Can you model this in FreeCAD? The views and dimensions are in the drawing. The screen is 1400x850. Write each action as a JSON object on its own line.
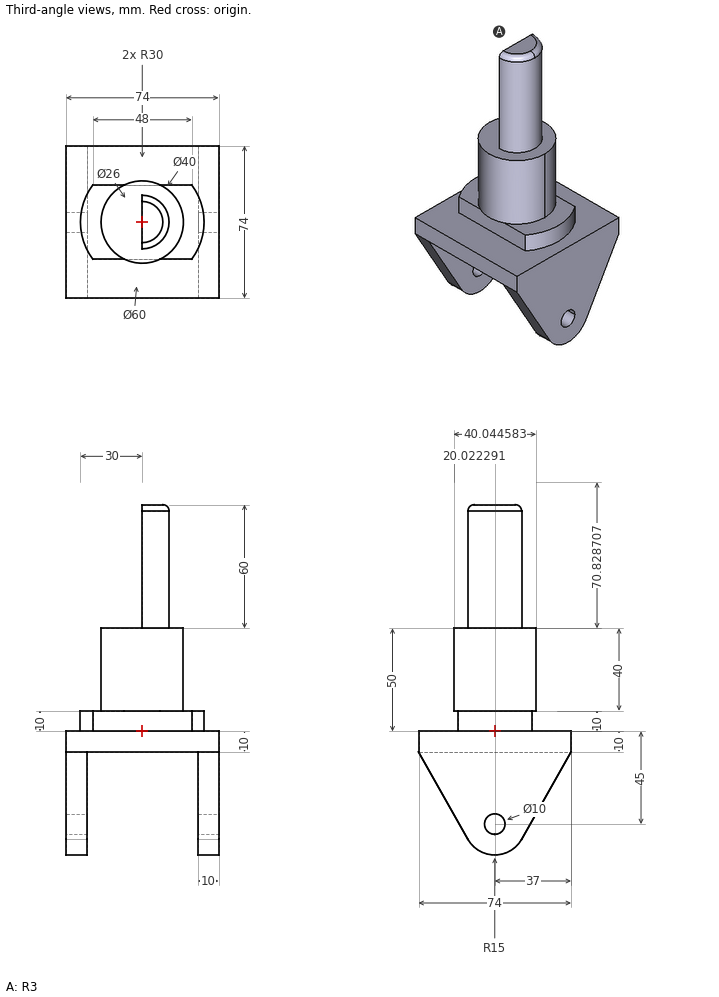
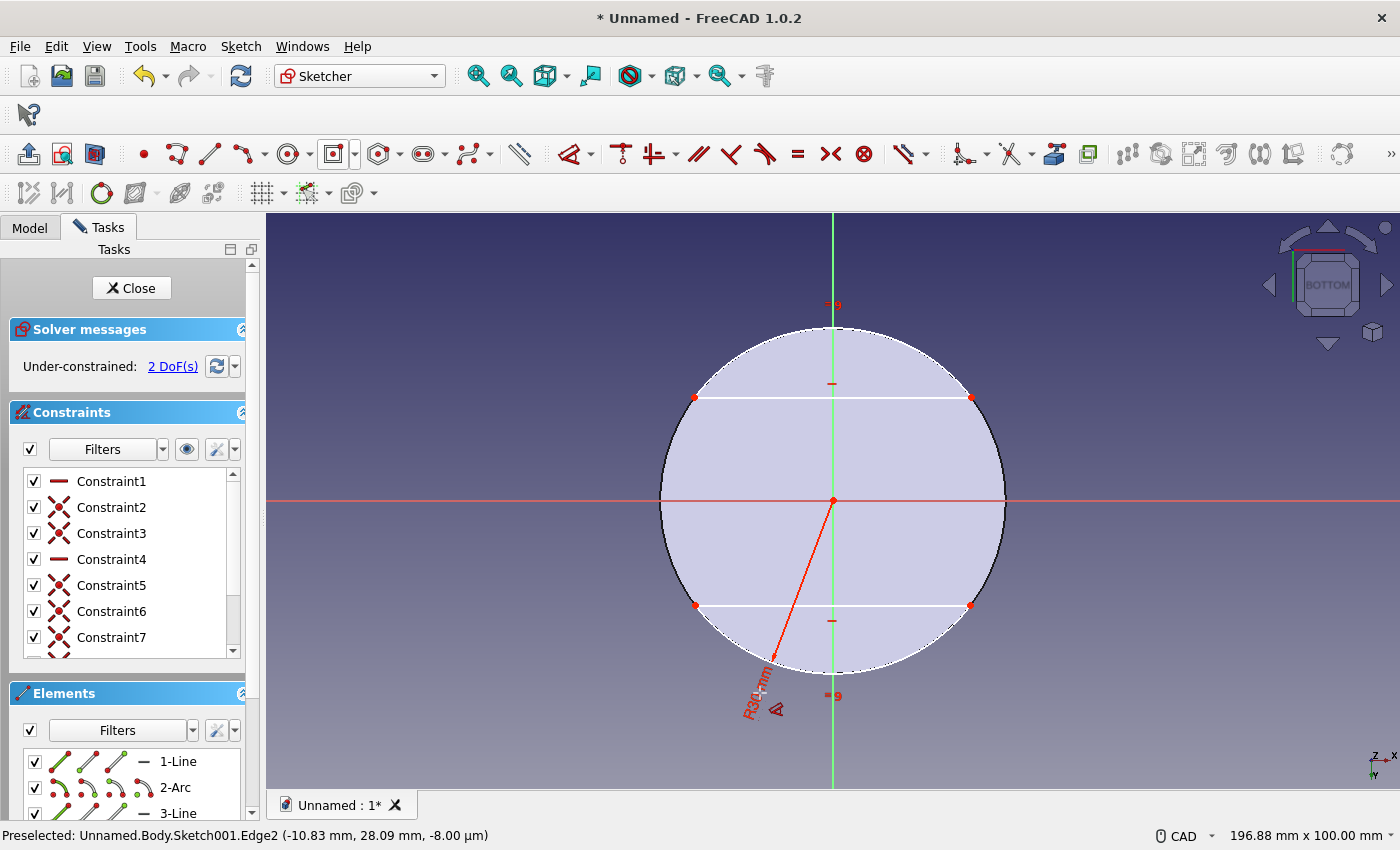
{"action": "left_click", "coordinate": [888, 606]}
{"action": "left_click", "coordinate": [770, 640]}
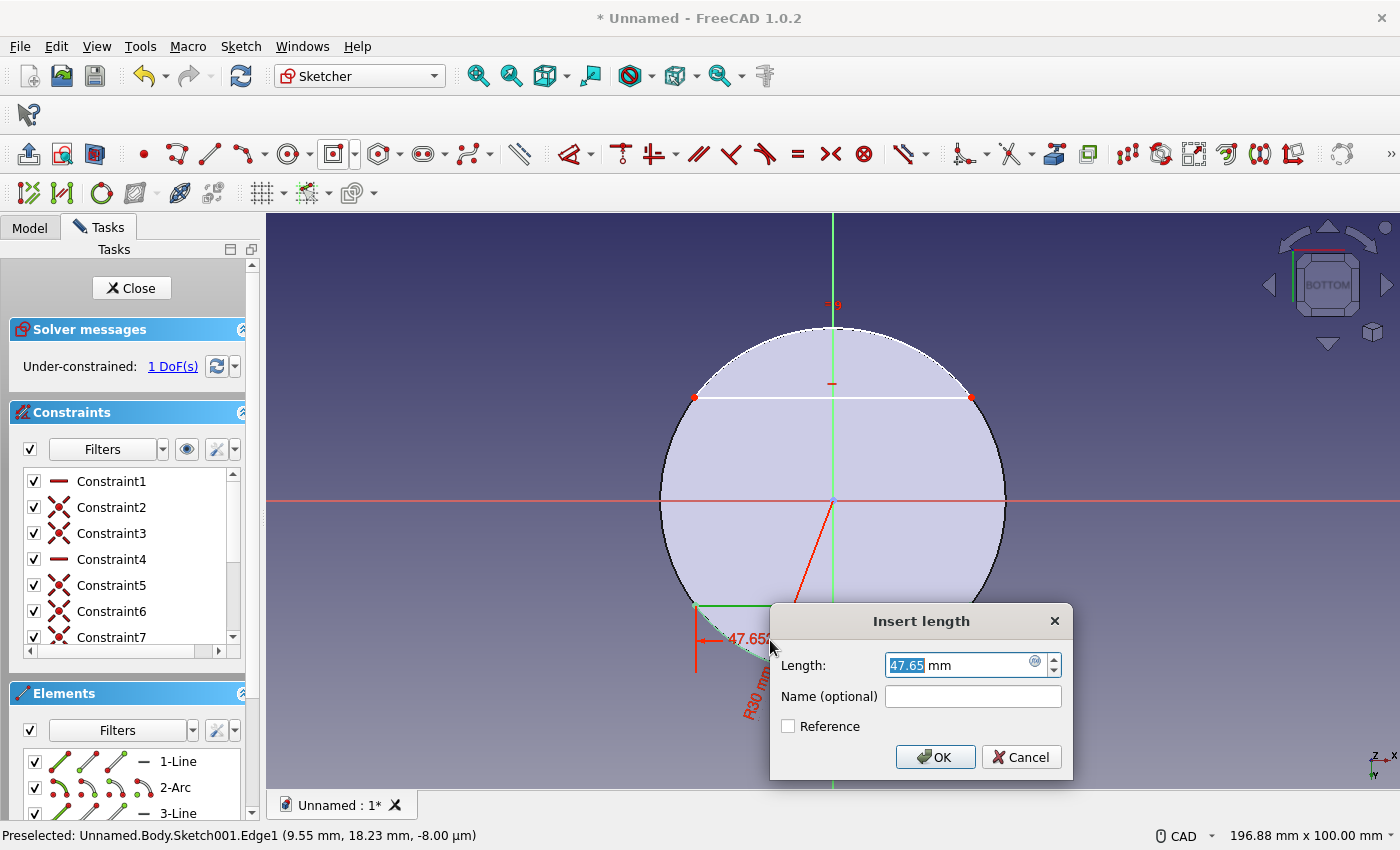
{"action": "type", "text": "48"}
{"action": "key", "text": "Return"}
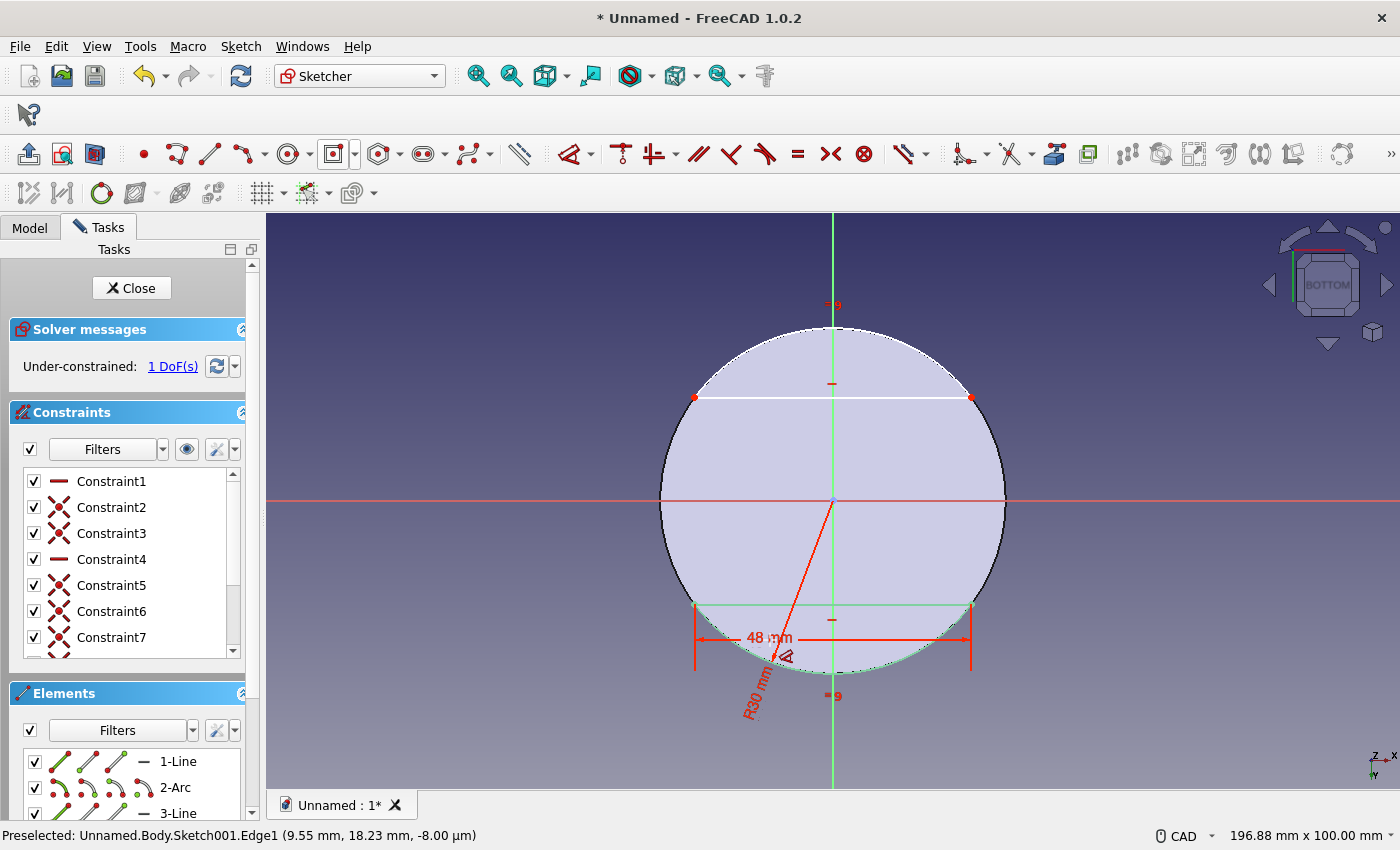
{"action": "left_click", "coordinate": [778, 398]}
{"action": "left_click", "coordinate": [769, 364]}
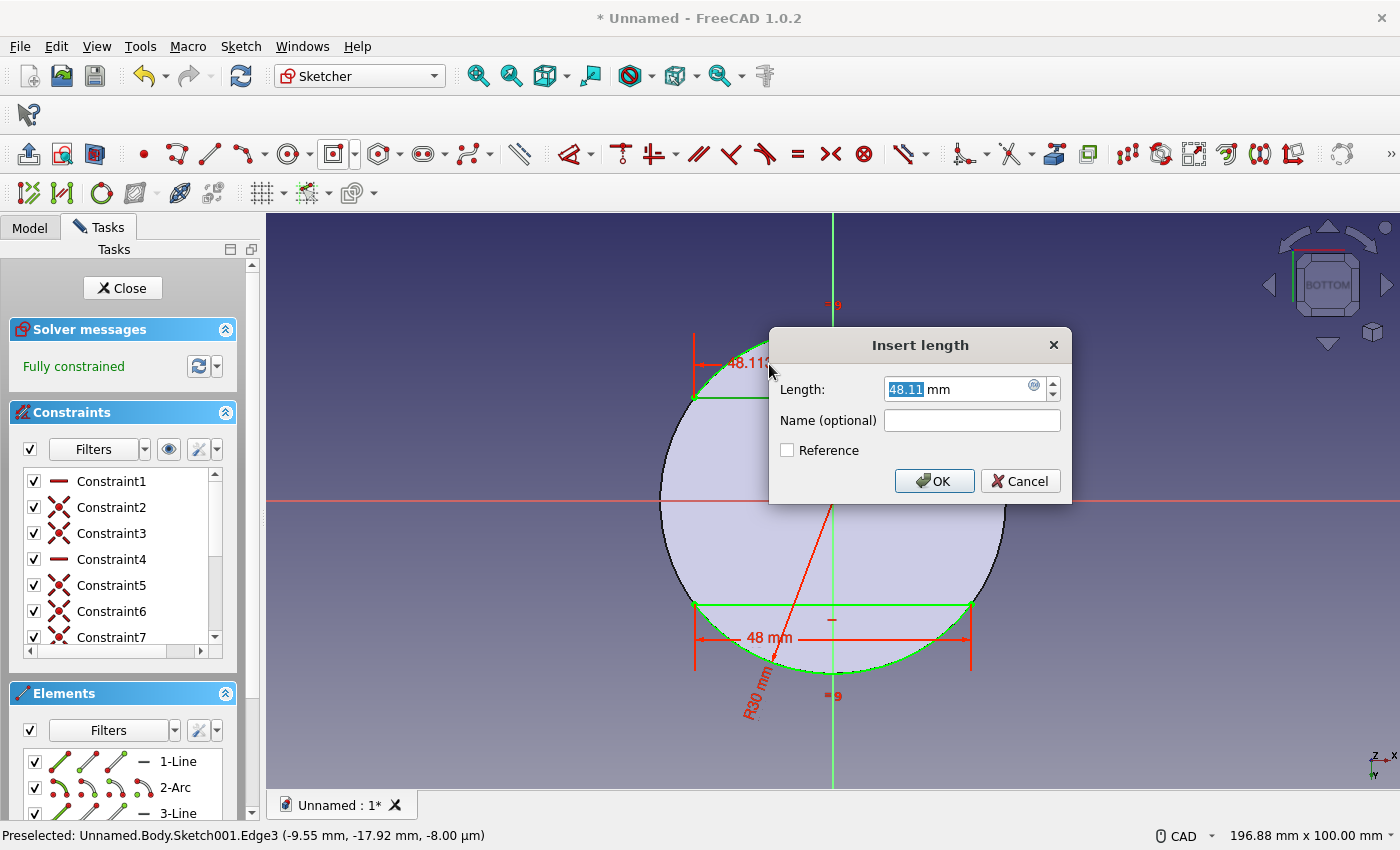
{"action": "type", "text": "48"}
{"action": "key", "text": "Return"}
{"action": "key", "text": "Escape"}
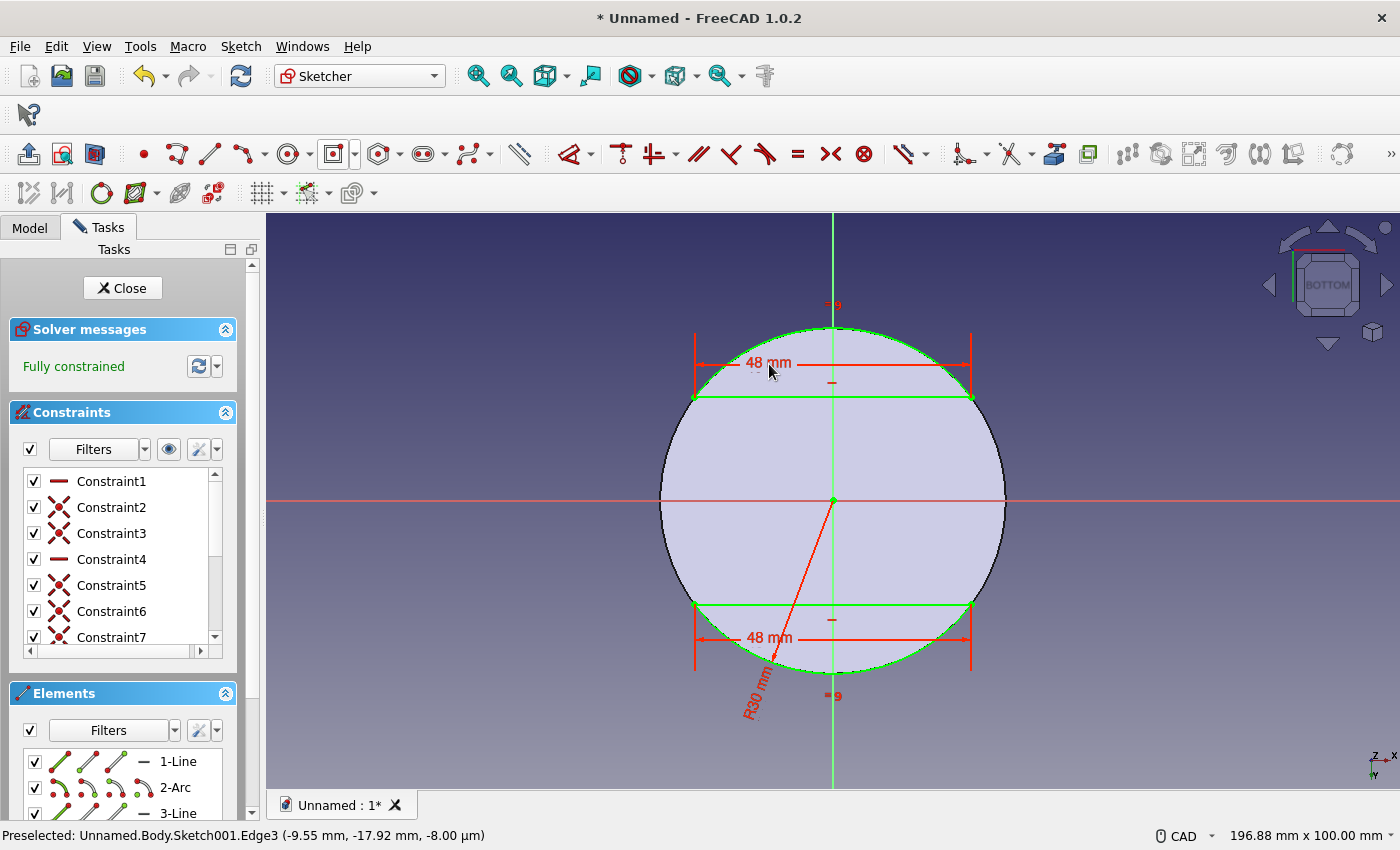
{"action": "left_click", "coordinate": [123, 288]}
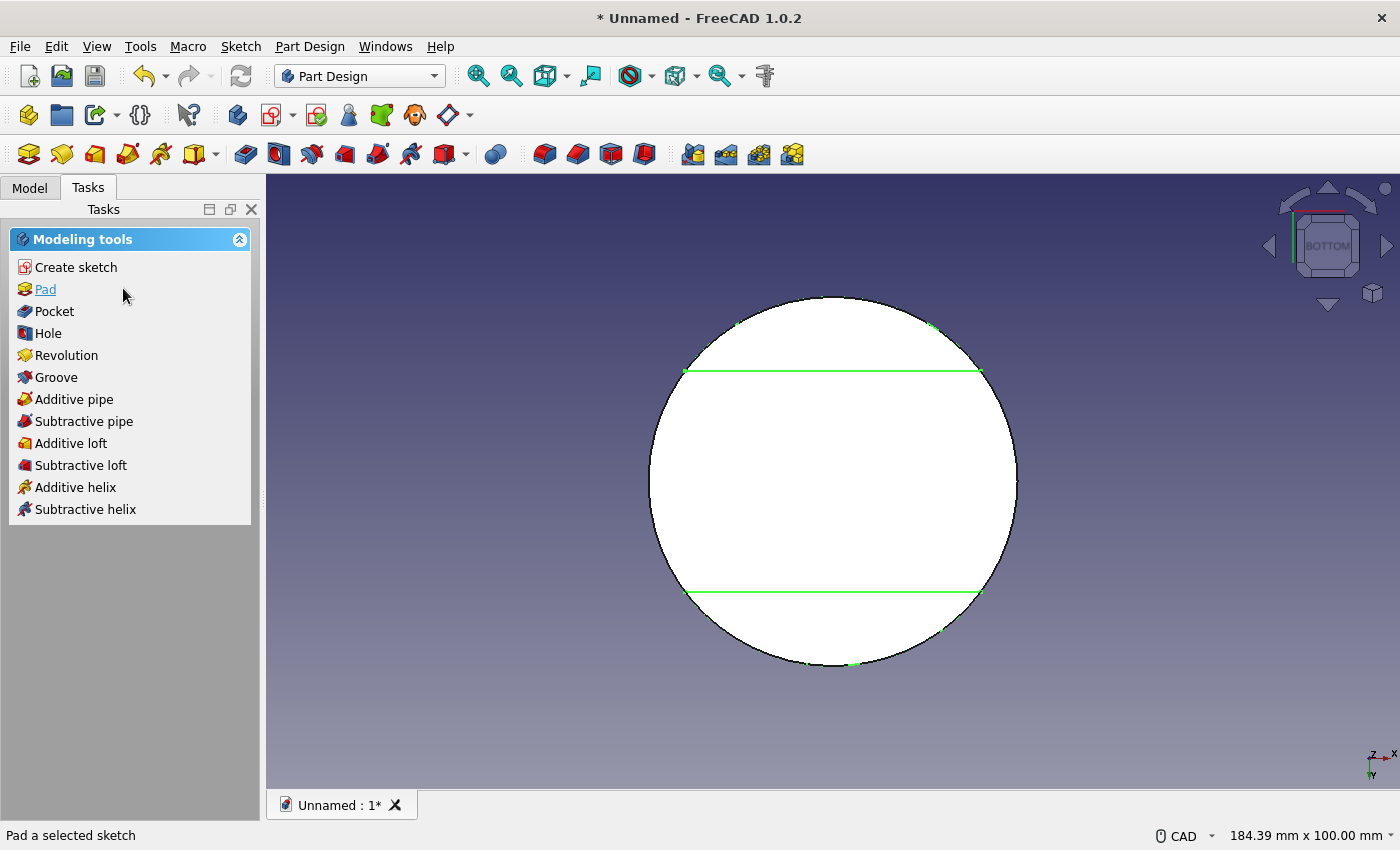
{"action": "left_click", "coordinate": [246, 154]}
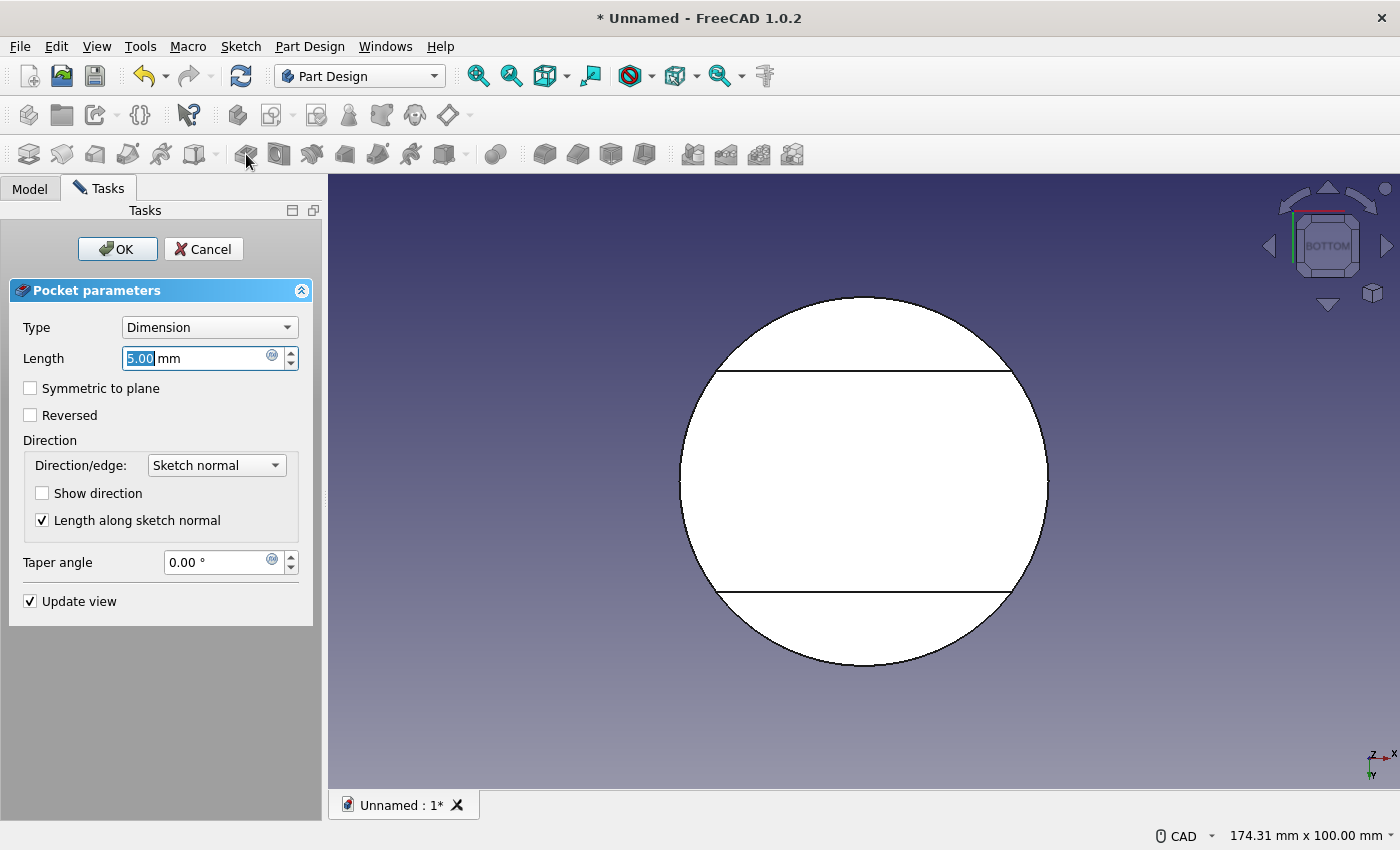
{"action": "type", "text": "10"}
{"action": "key", "text": "Tab"}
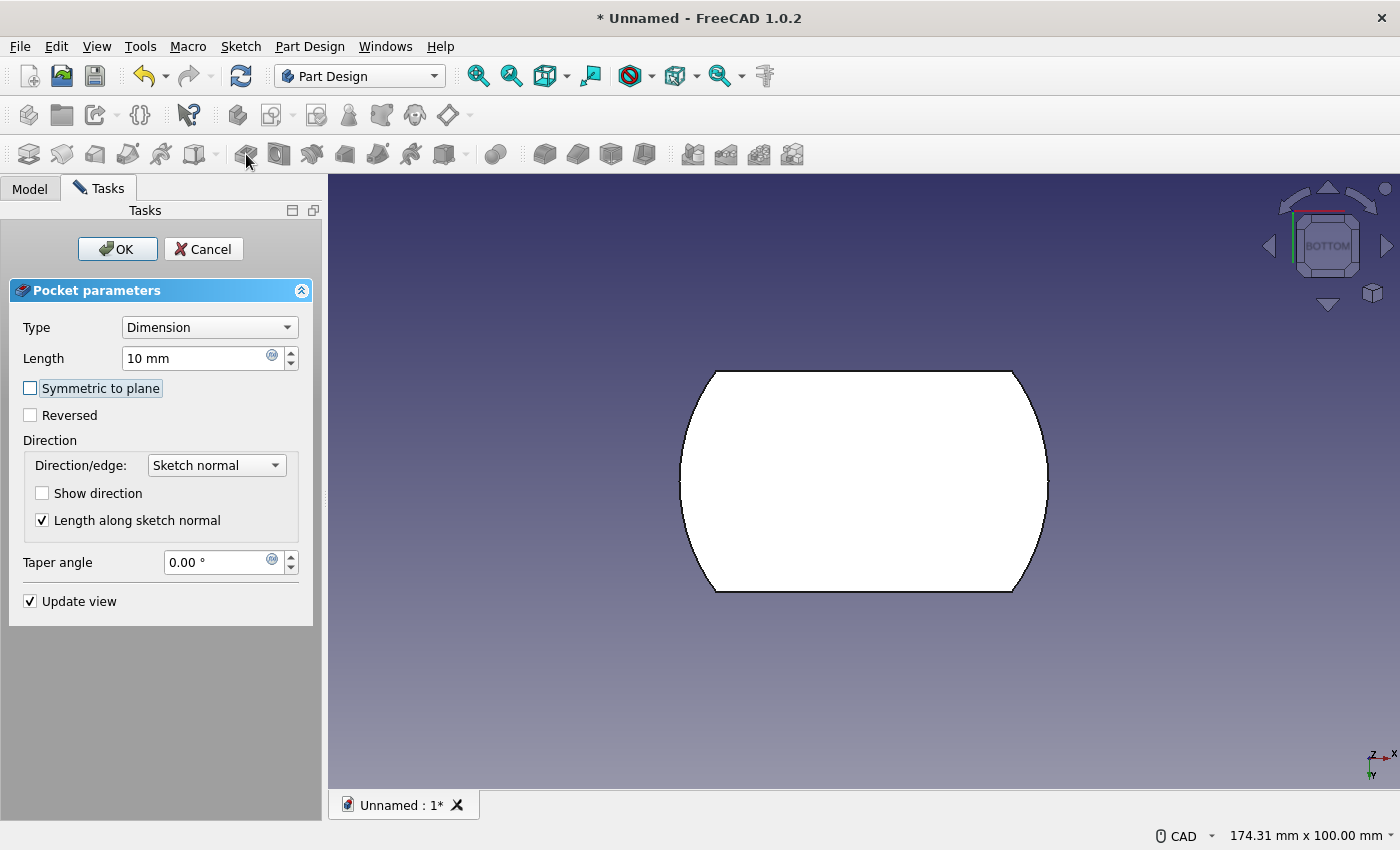
{"action": "left_click", "coordinate": [118, 249]}